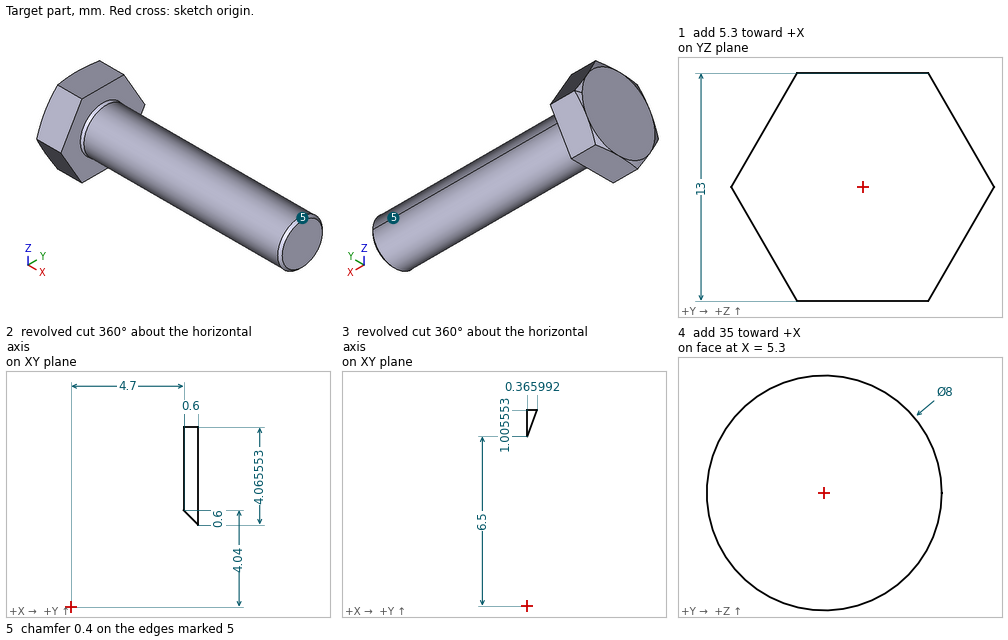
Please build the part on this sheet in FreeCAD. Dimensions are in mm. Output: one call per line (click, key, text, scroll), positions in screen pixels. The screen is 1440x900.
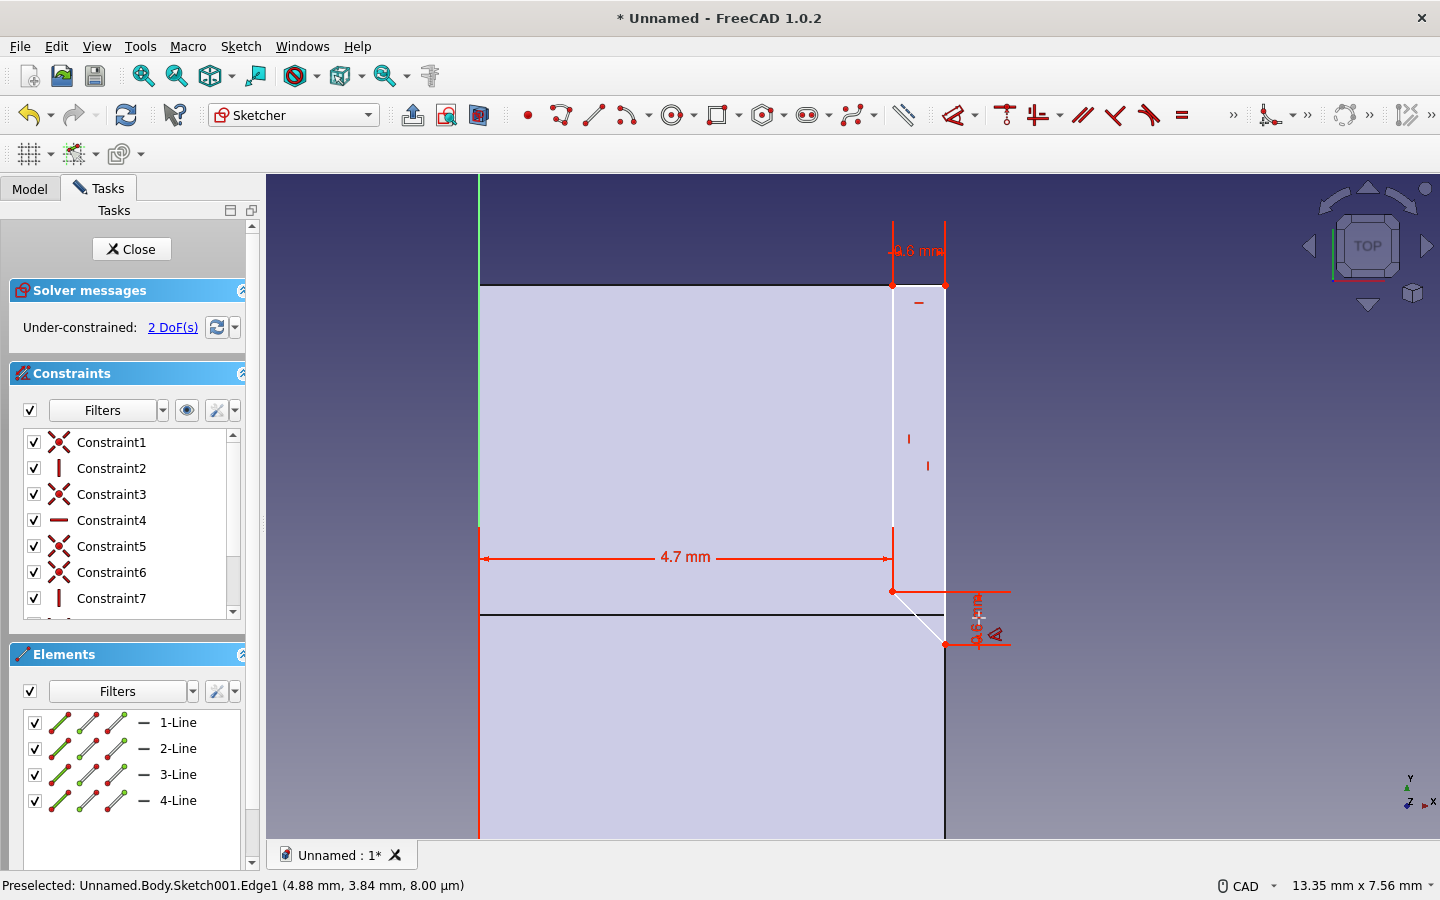
click(893, 592)
click(445, 701)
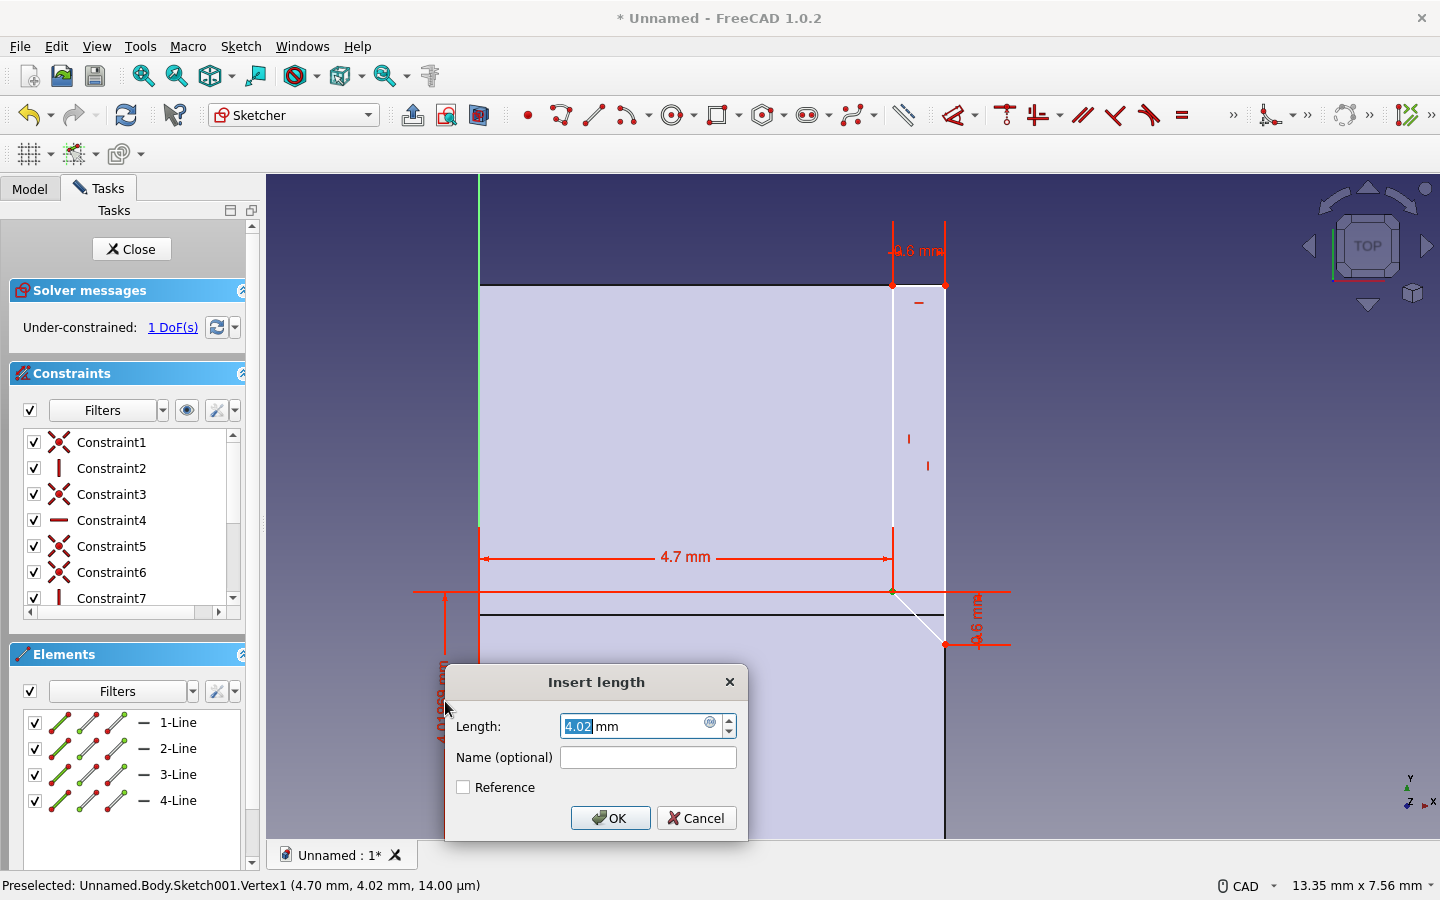
text(4.04)
key(Return)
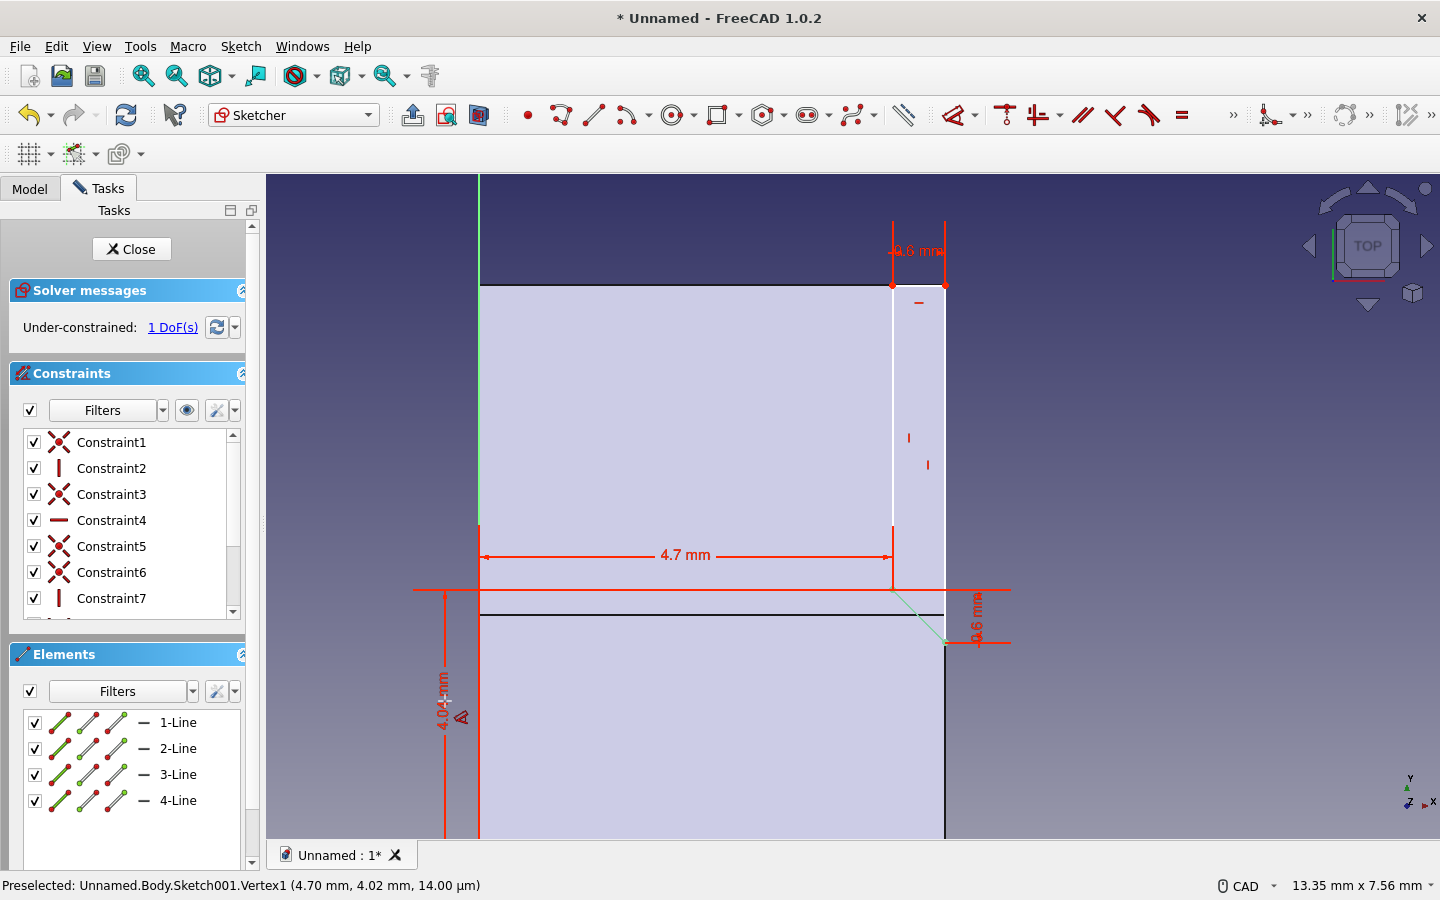
click(945, 536)
click(979, 464)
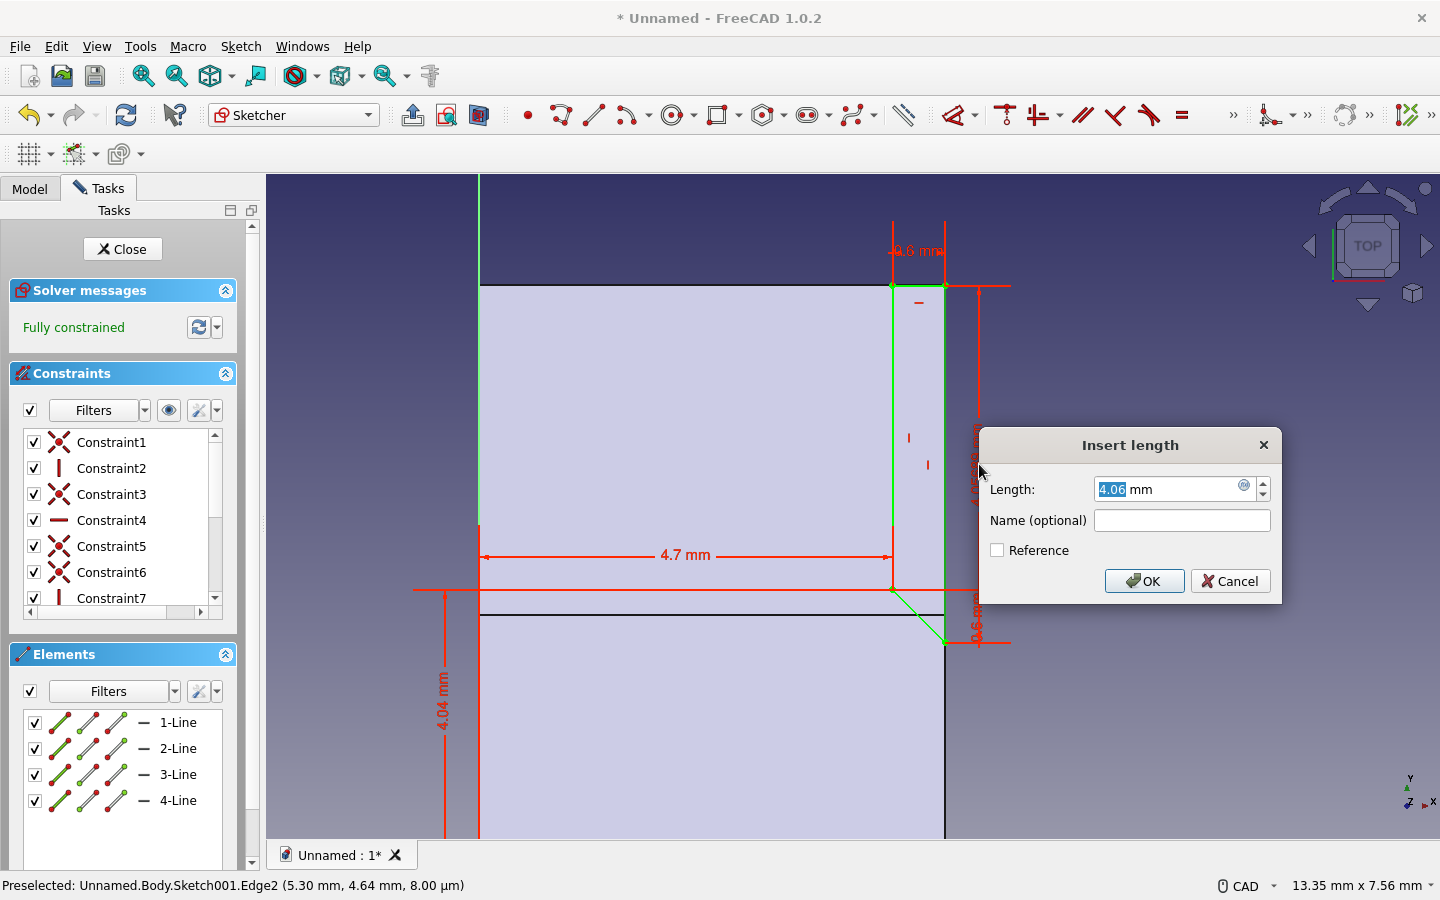
text(4.065553)
key(Return)
key(Escape)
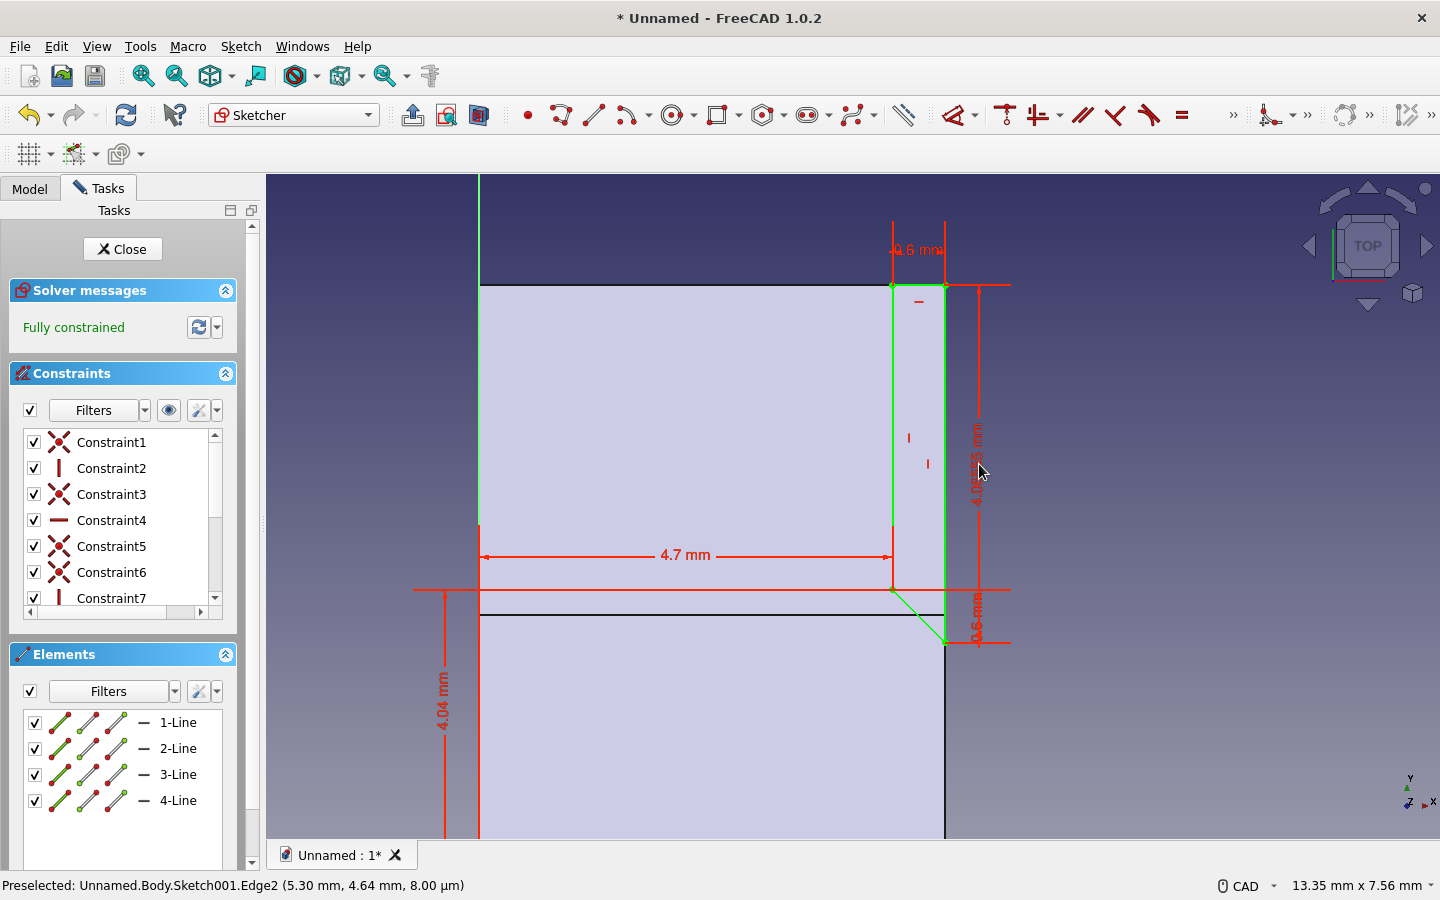
click(123, 249)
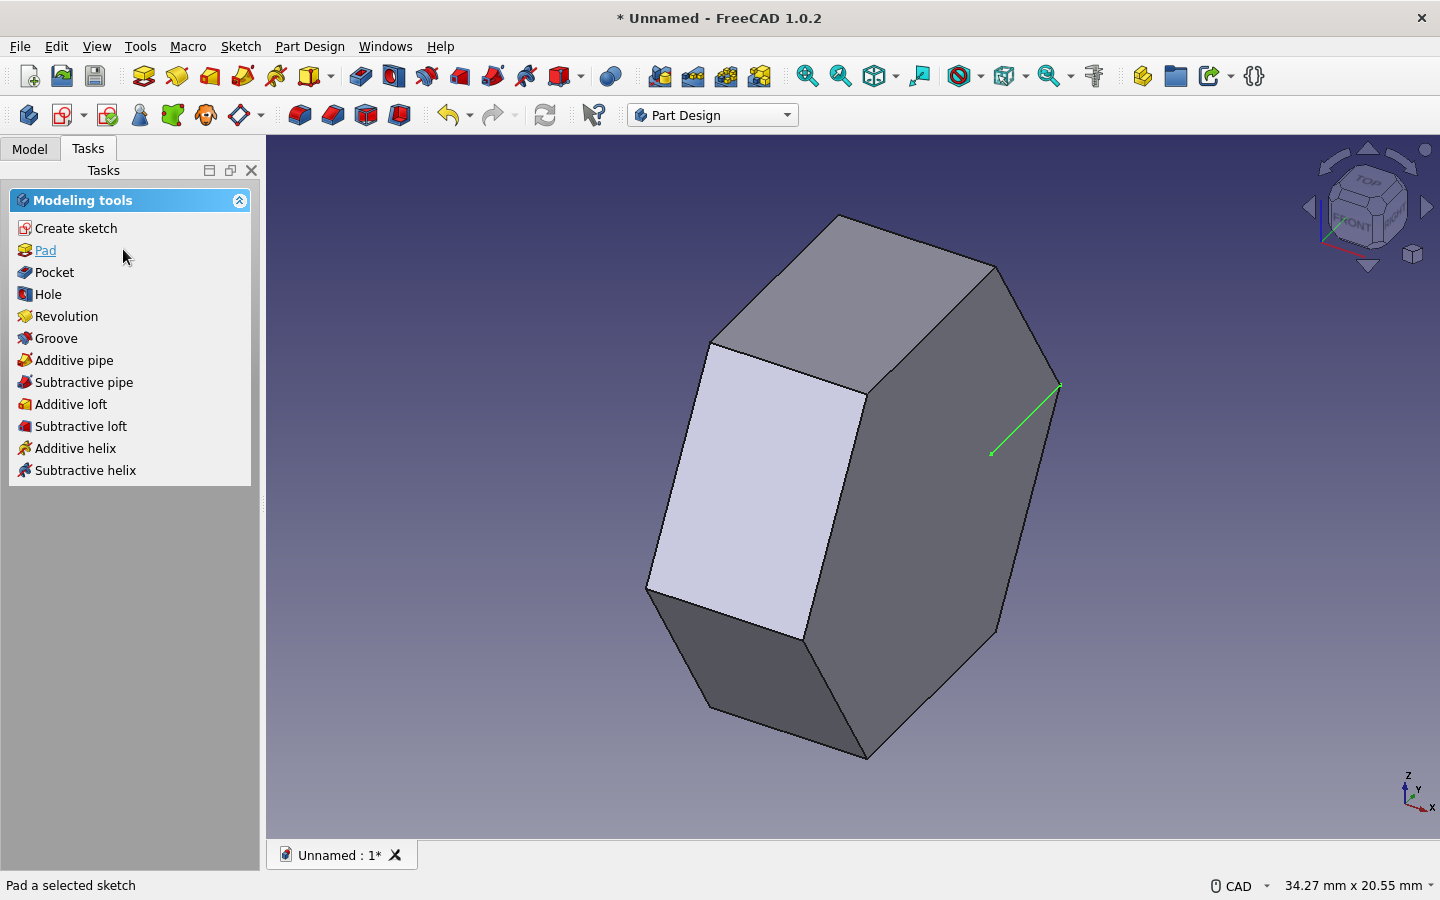
click(427, 76)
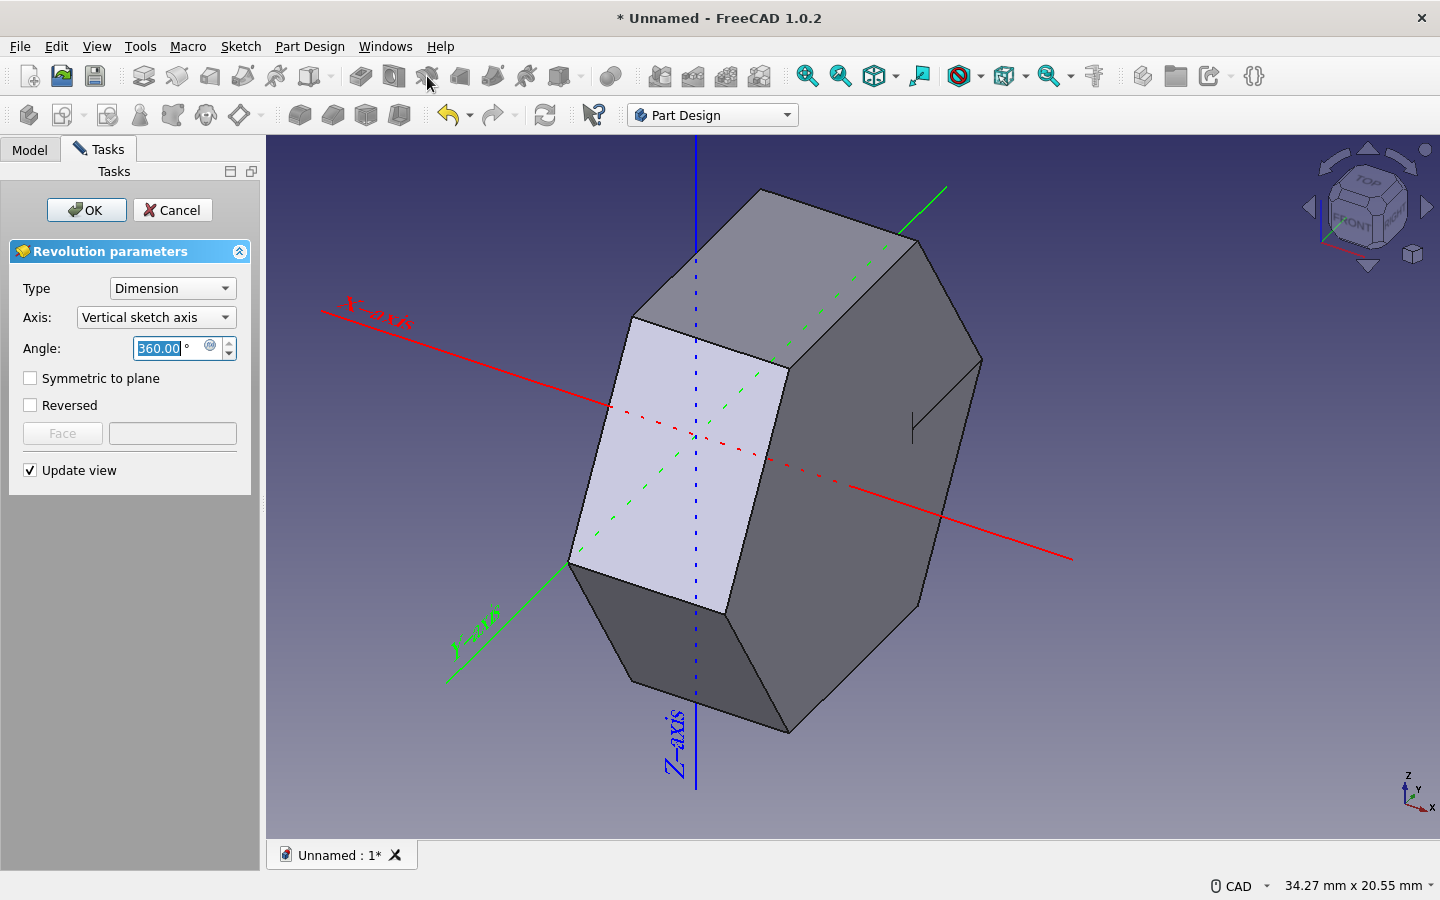
click(157, 318)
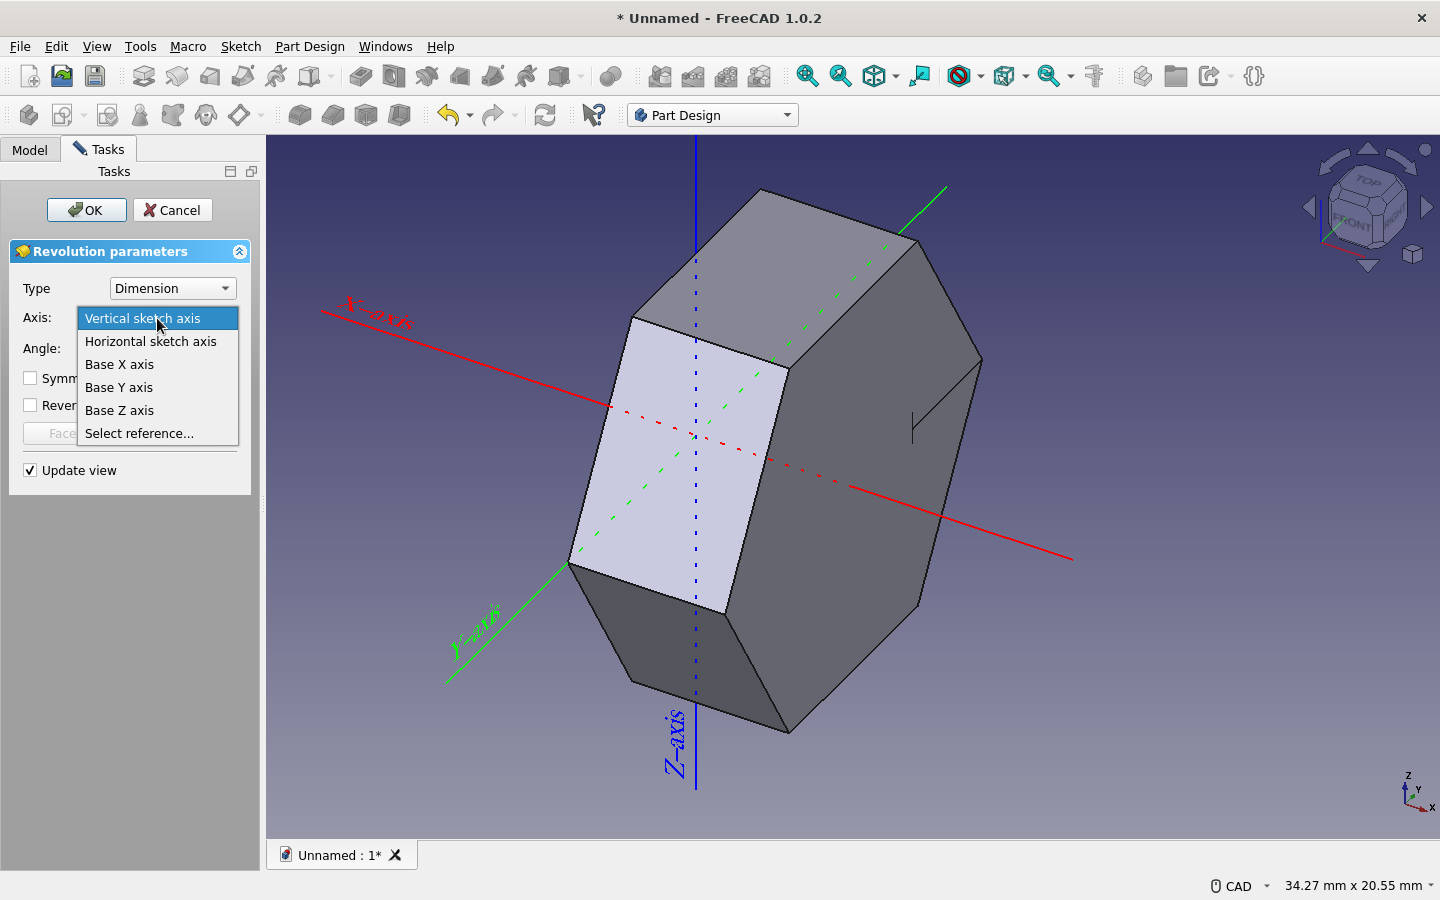
click(156, 342)